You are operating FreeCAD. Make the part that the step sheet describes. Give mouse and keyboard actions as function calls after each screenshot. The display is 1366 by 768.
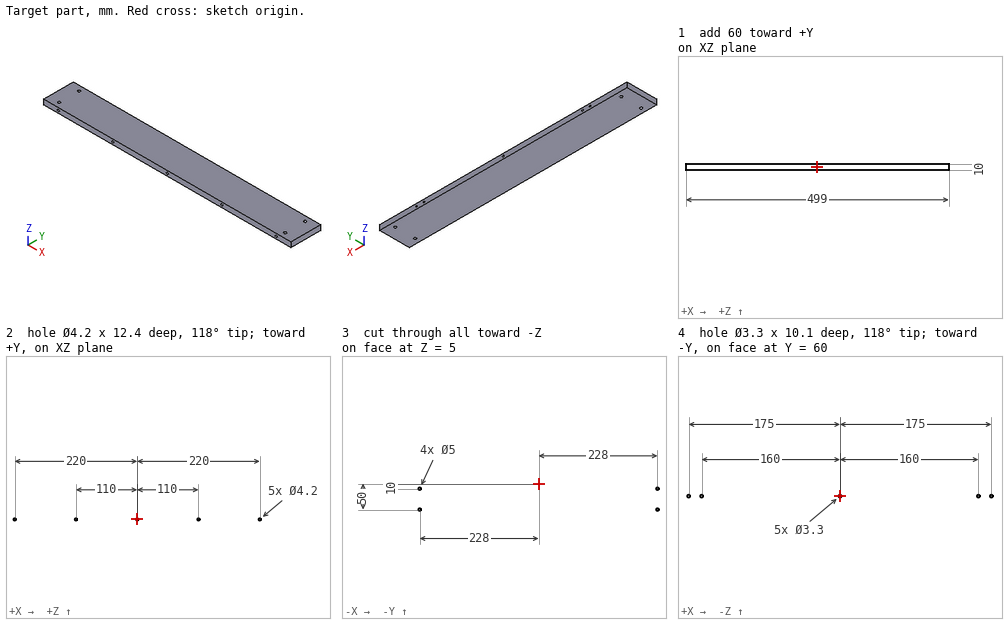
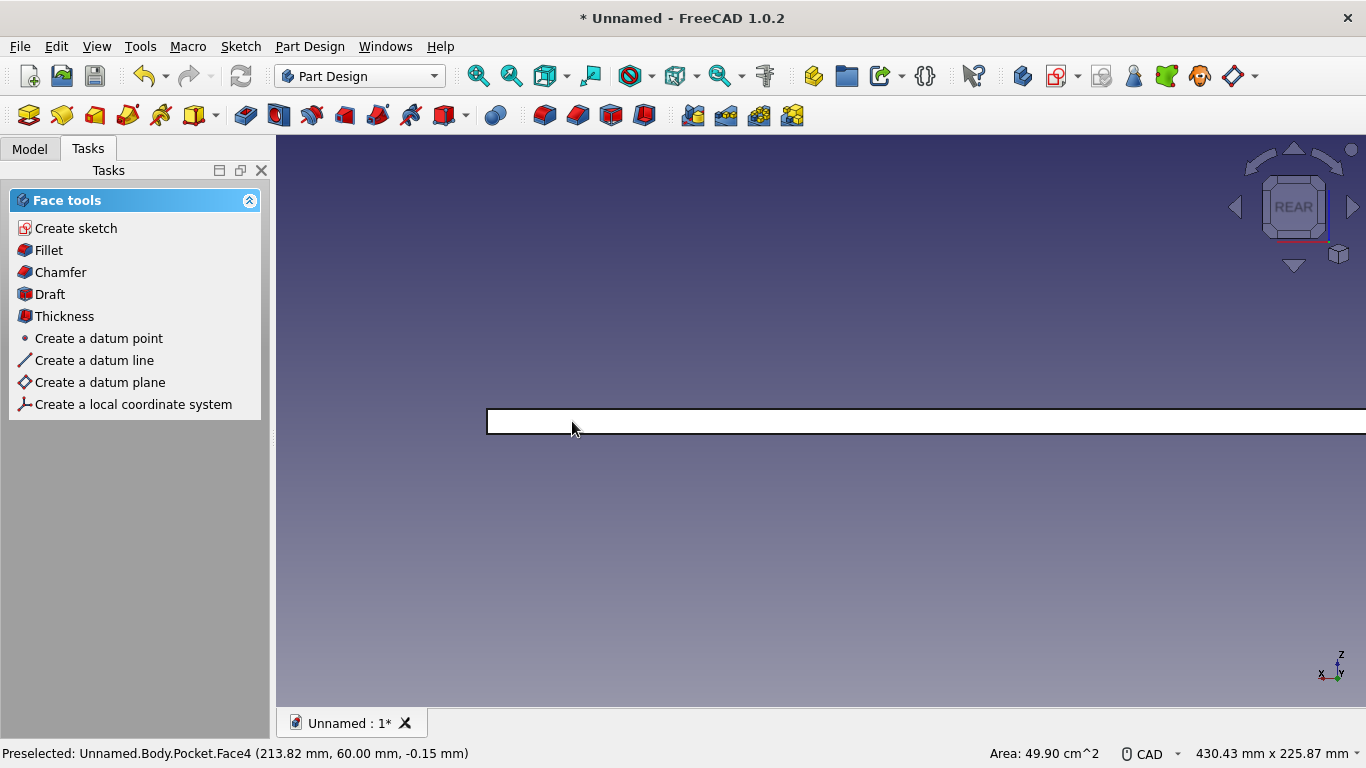
click(1056, 76)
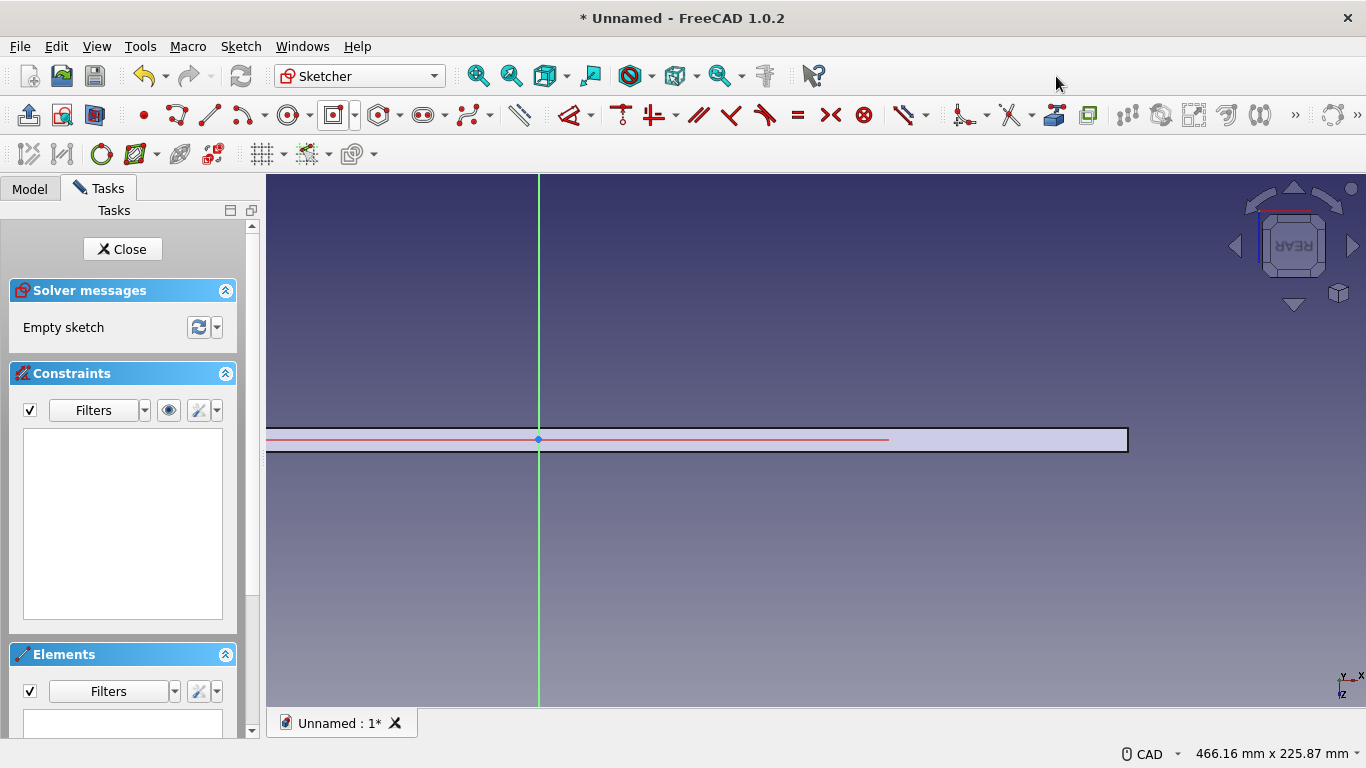
scroll(1172, 442, down, 2)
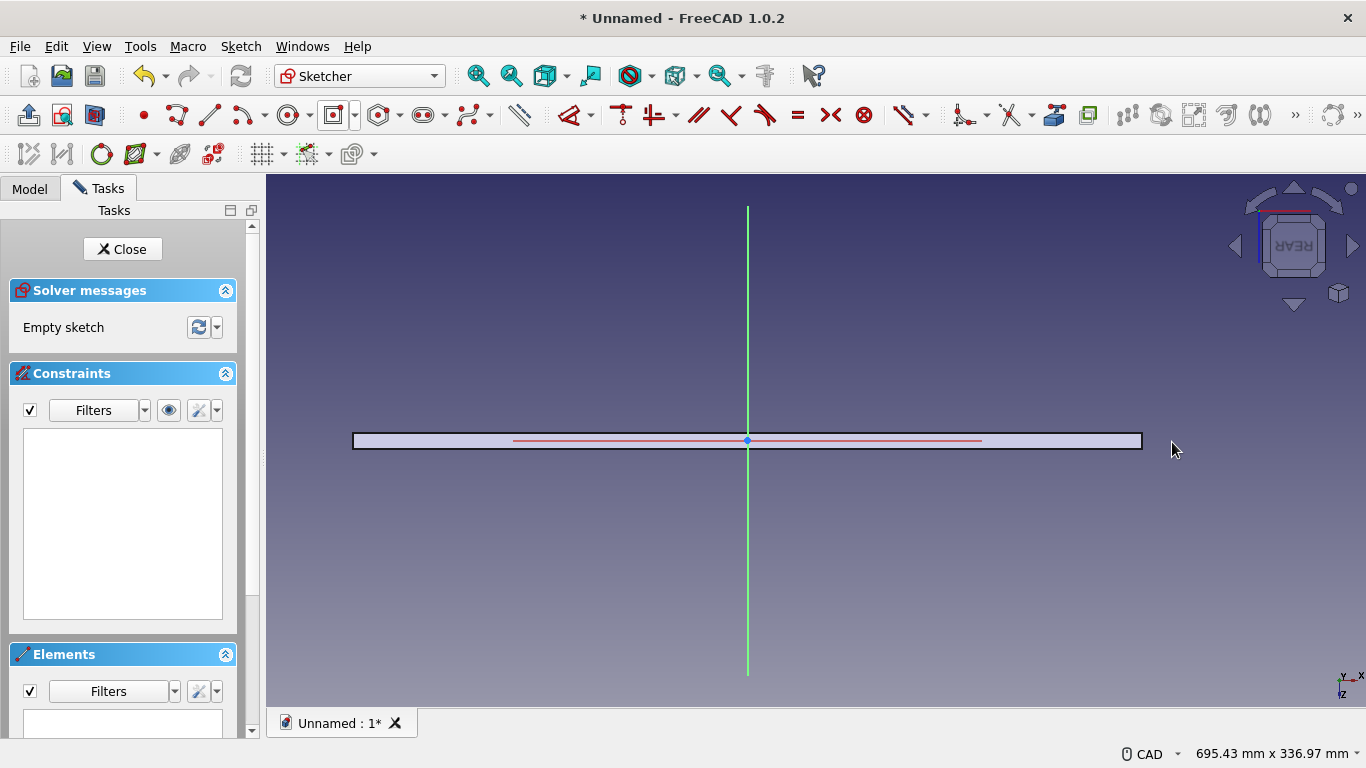
key(g)
key(c)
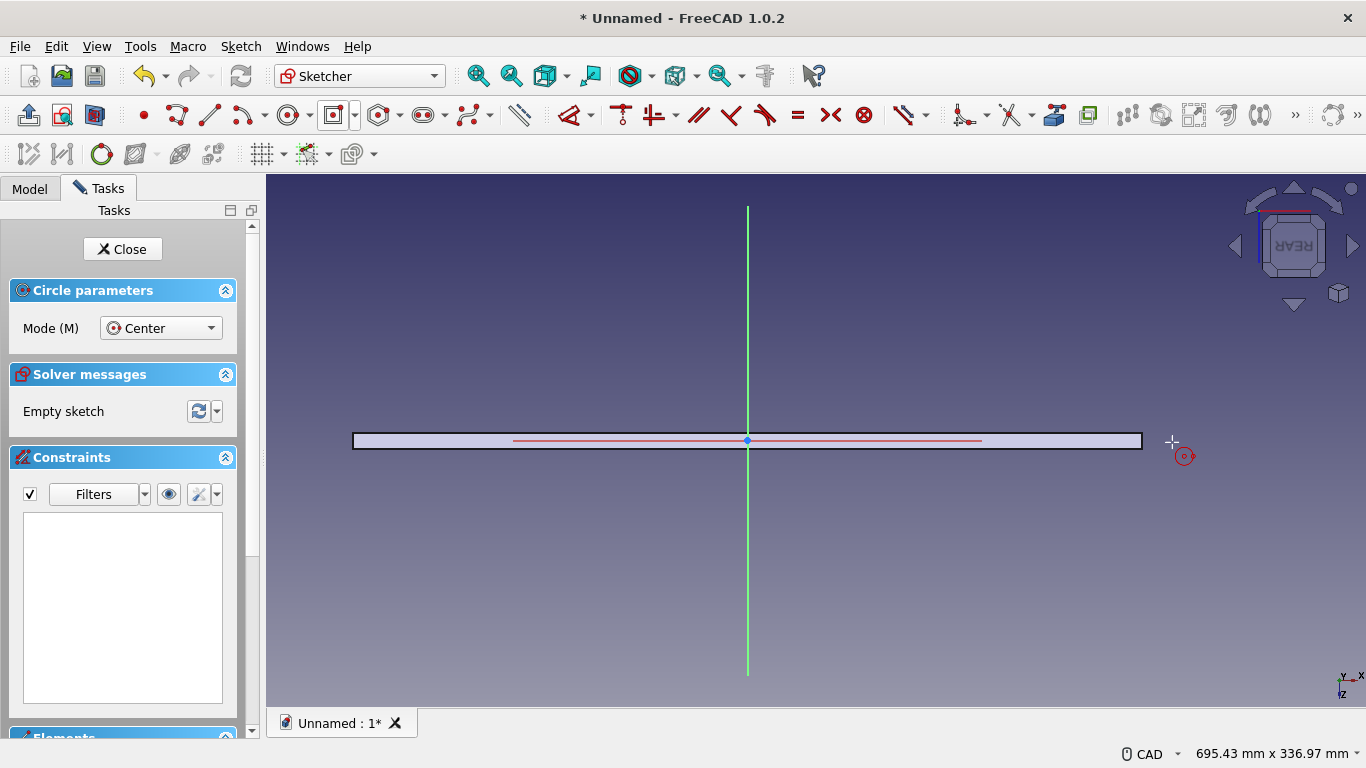
scroll(748, 441, up, 11)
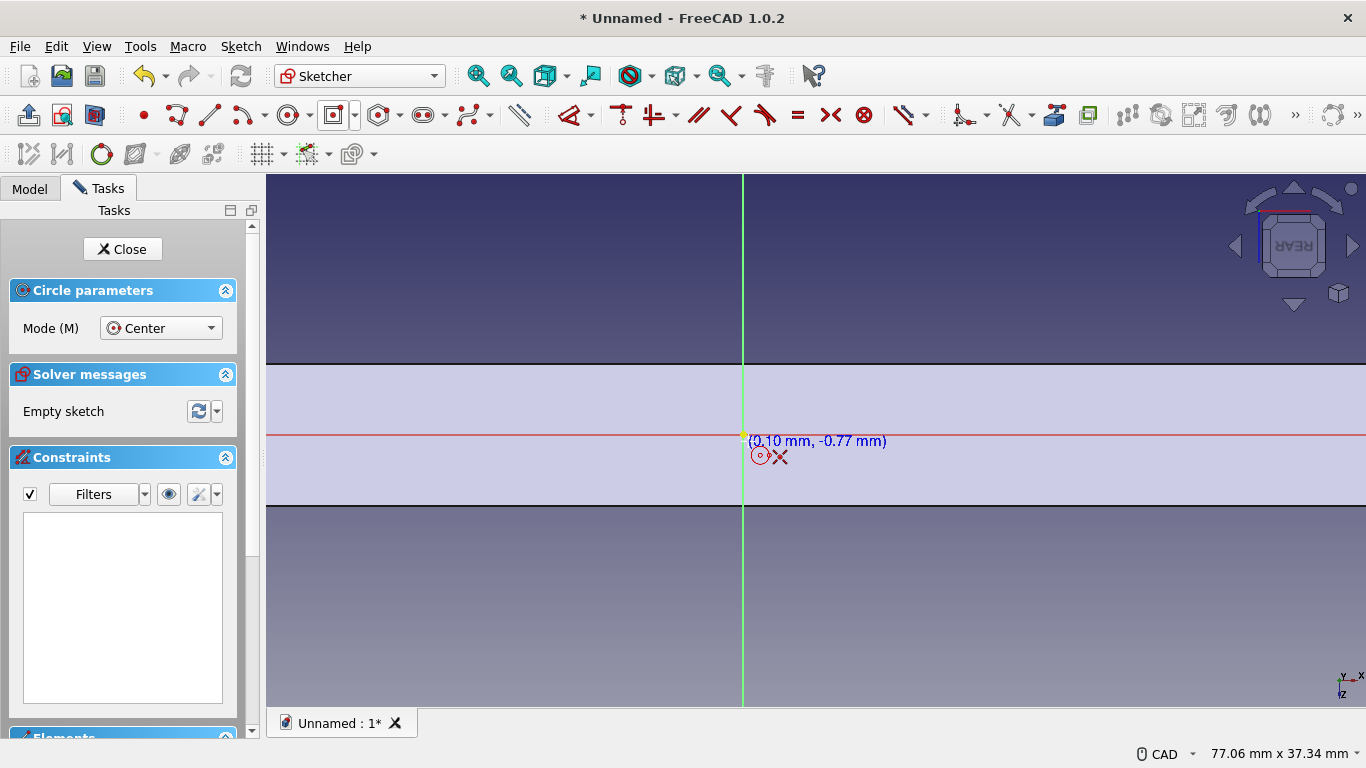
scroll(748, 441, down, 10)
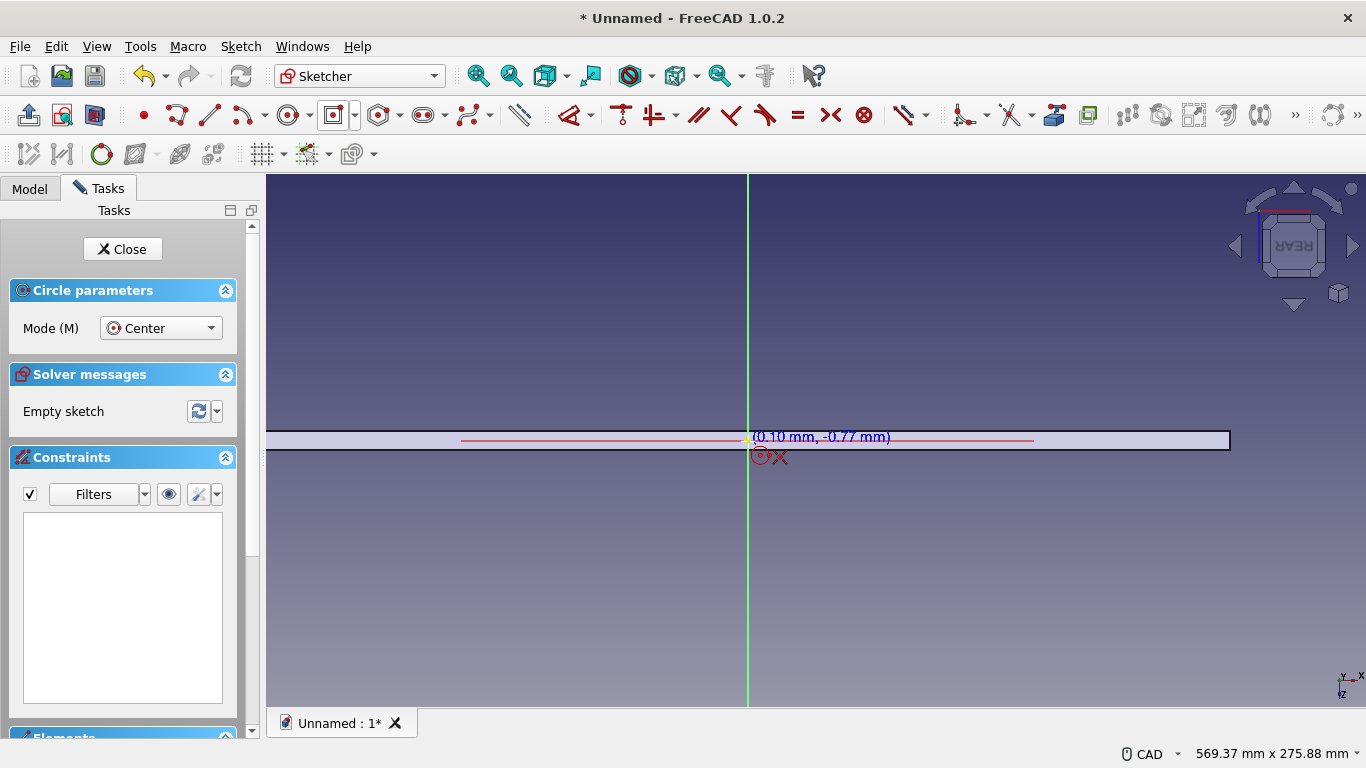
click(748, 441)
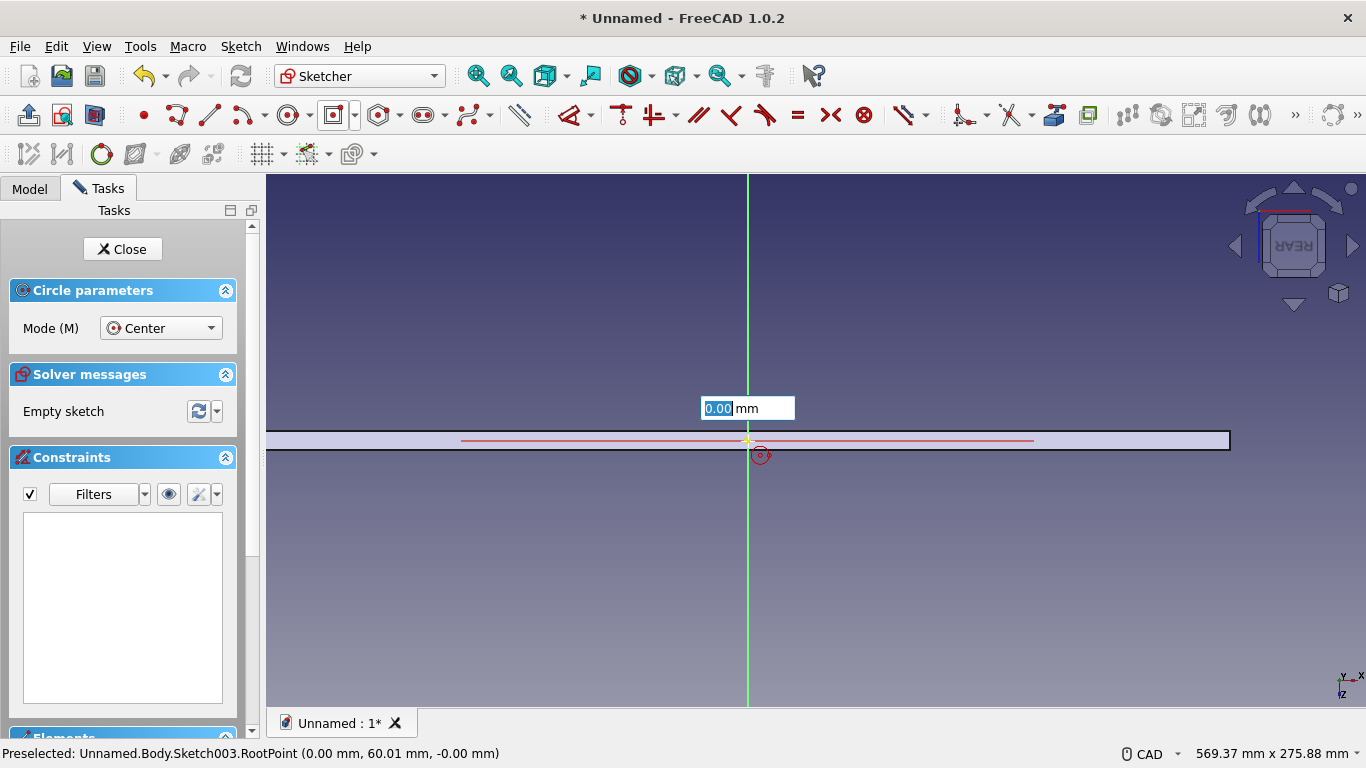
scroll(750, 438, up, 10)
move(747, 438)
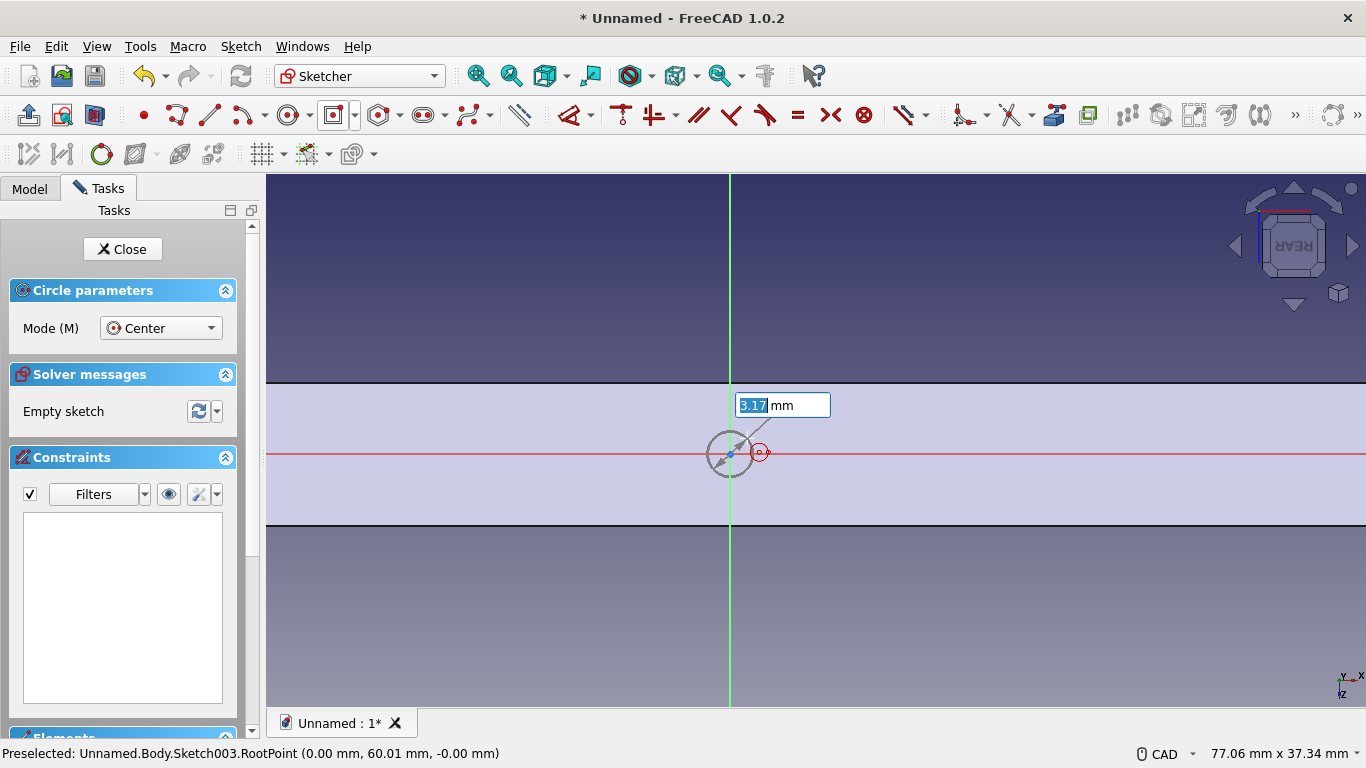
text(3.3)
key(Return)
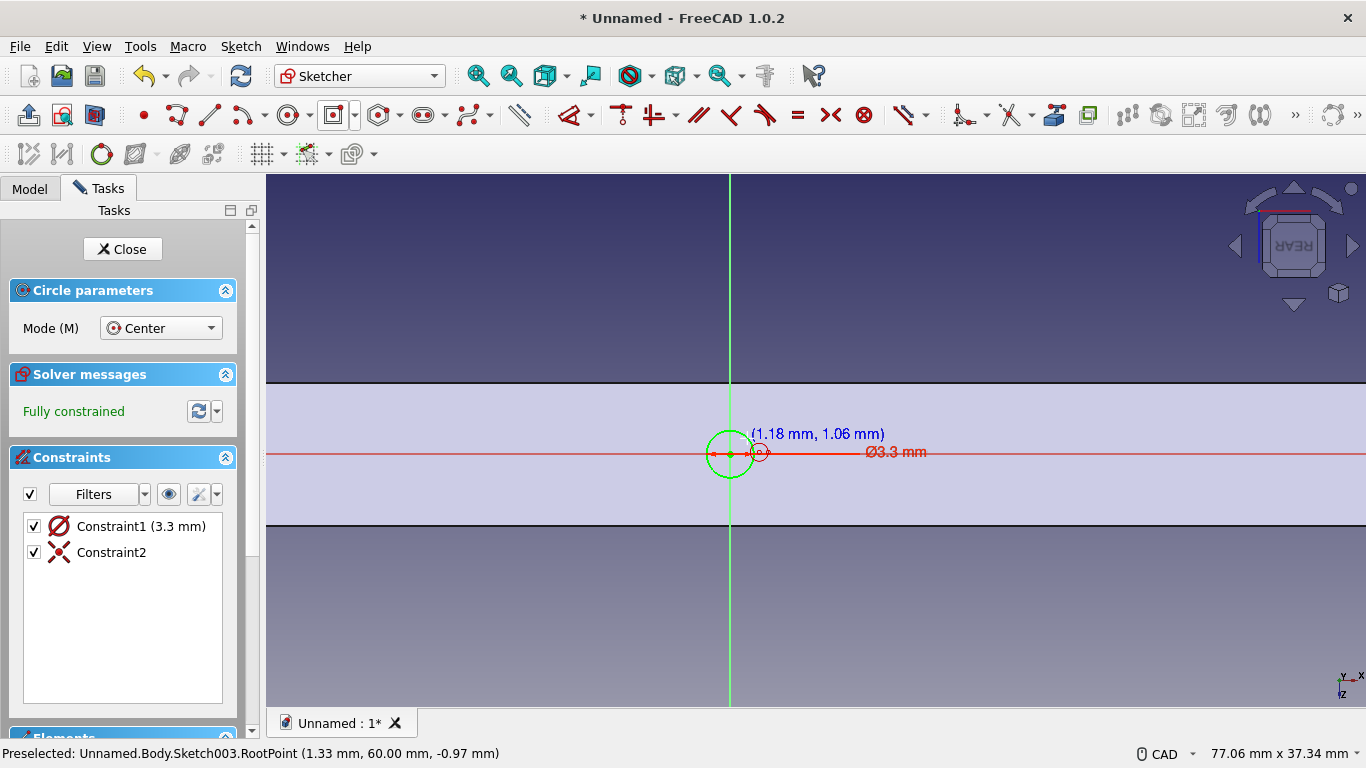
scroll(750, 438, down, 10)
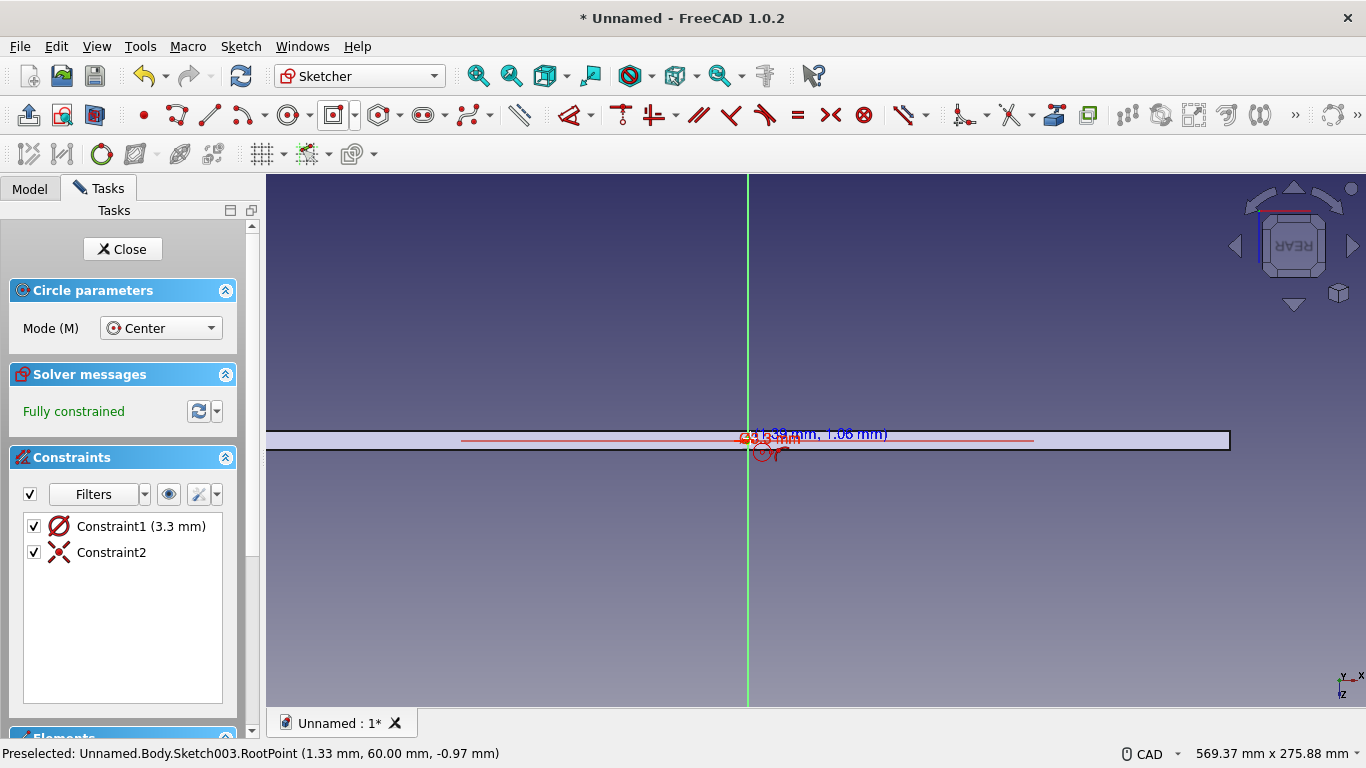
scroll(410, 441, up, 10)